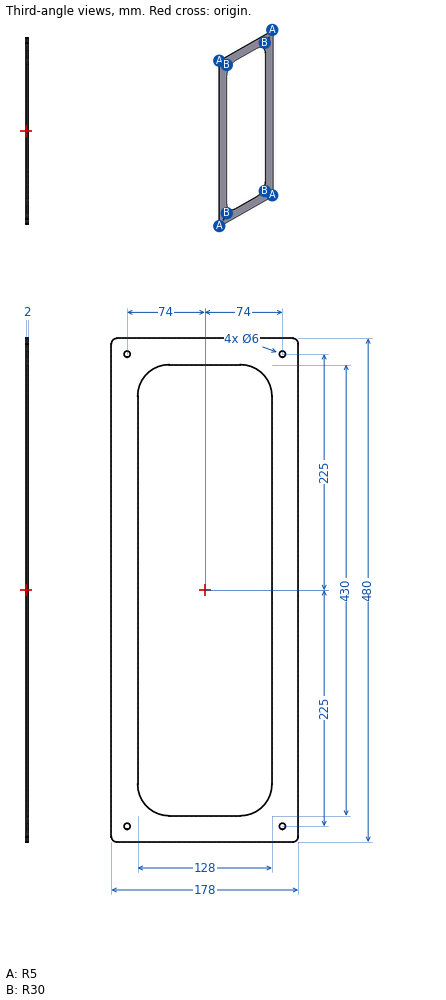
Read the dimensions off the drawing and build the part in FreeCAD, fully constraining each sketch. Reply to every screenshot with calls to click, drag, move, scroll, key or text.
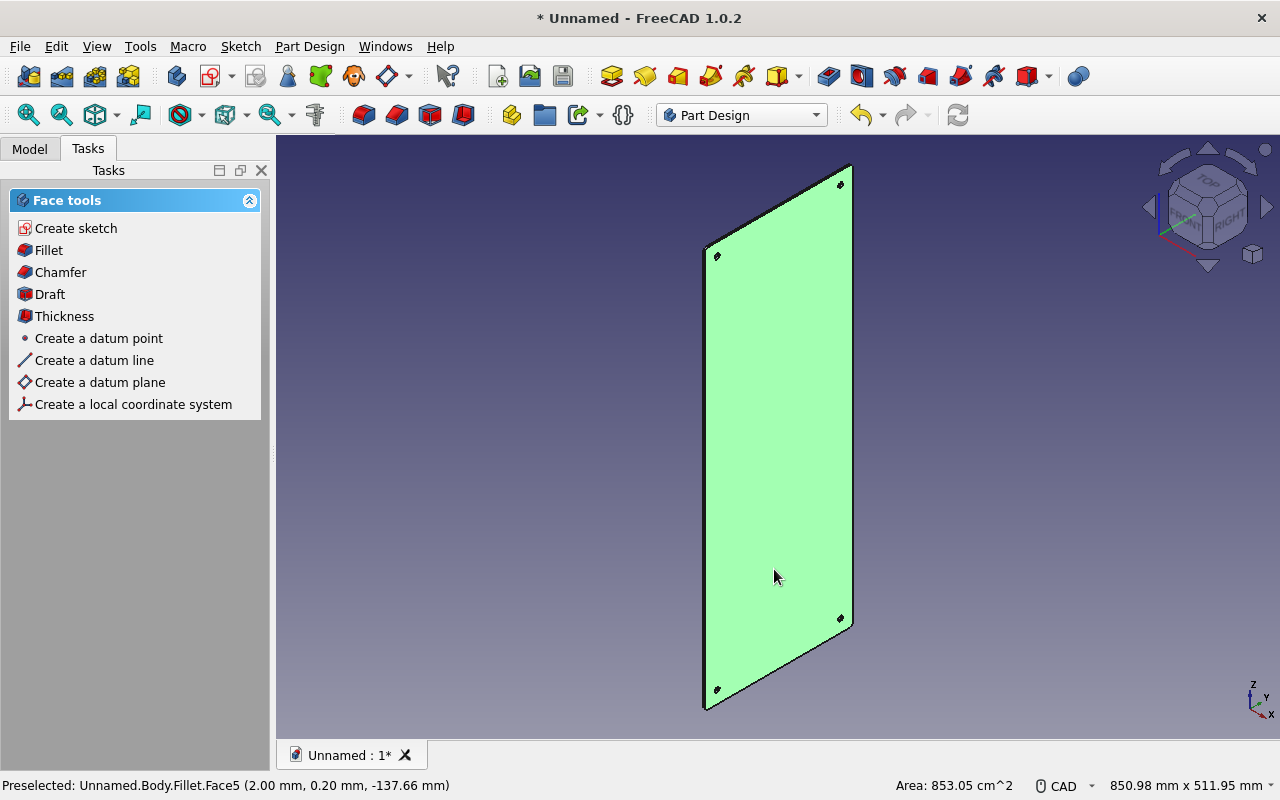
click(210, 76)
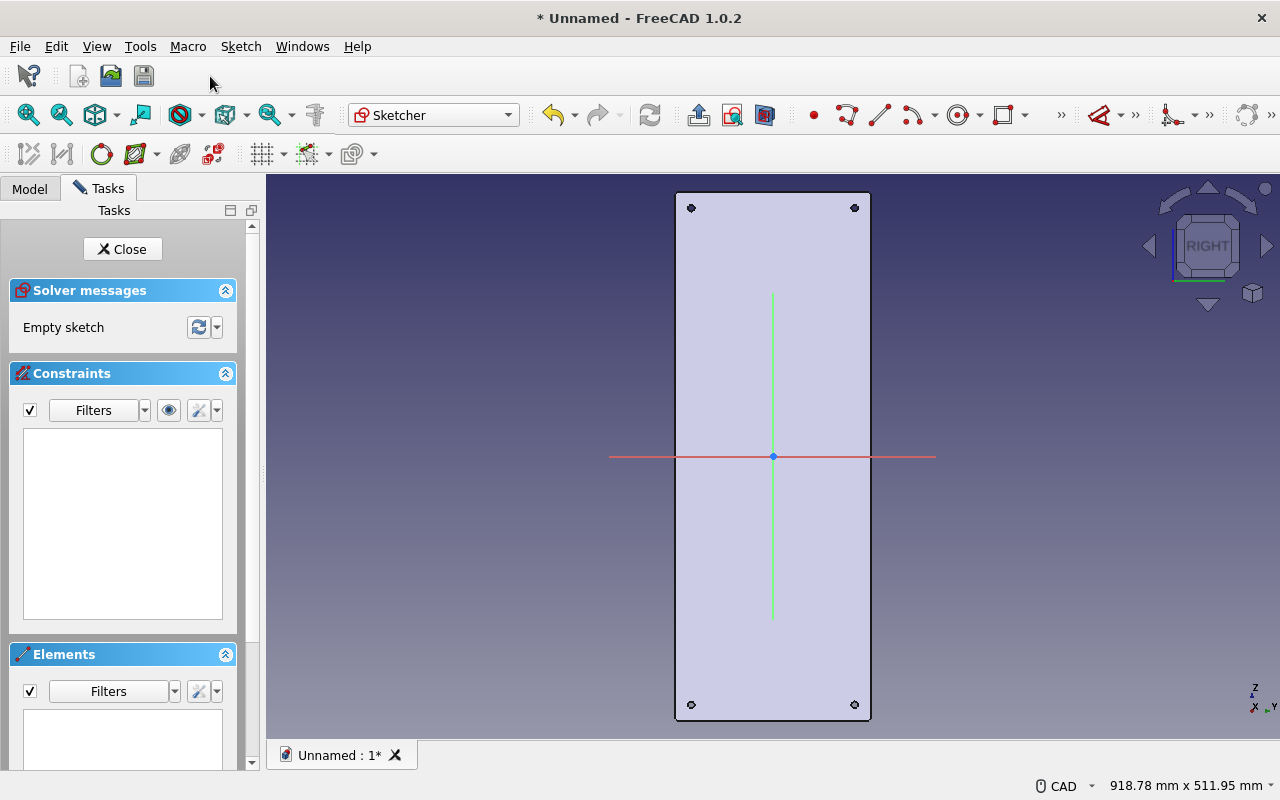
scroll(395, 456, down, 1)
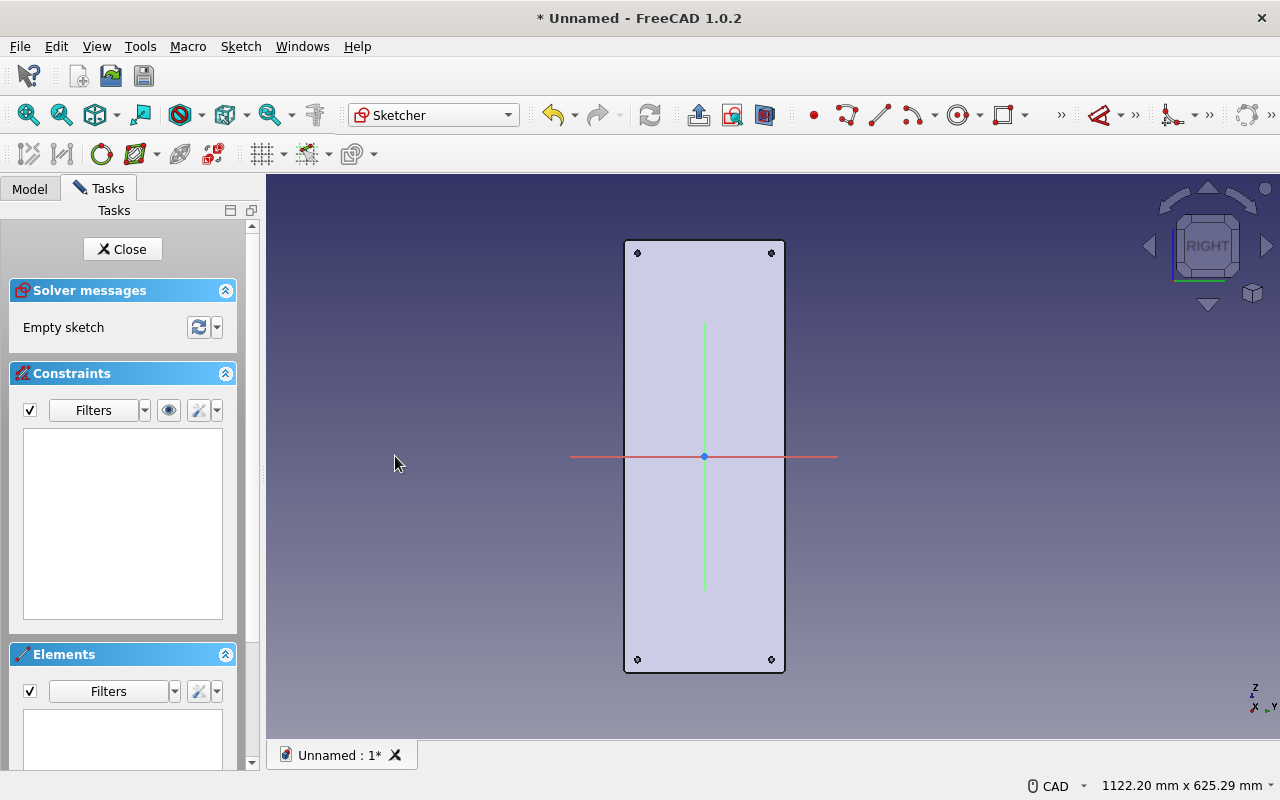
key(g)
key(v)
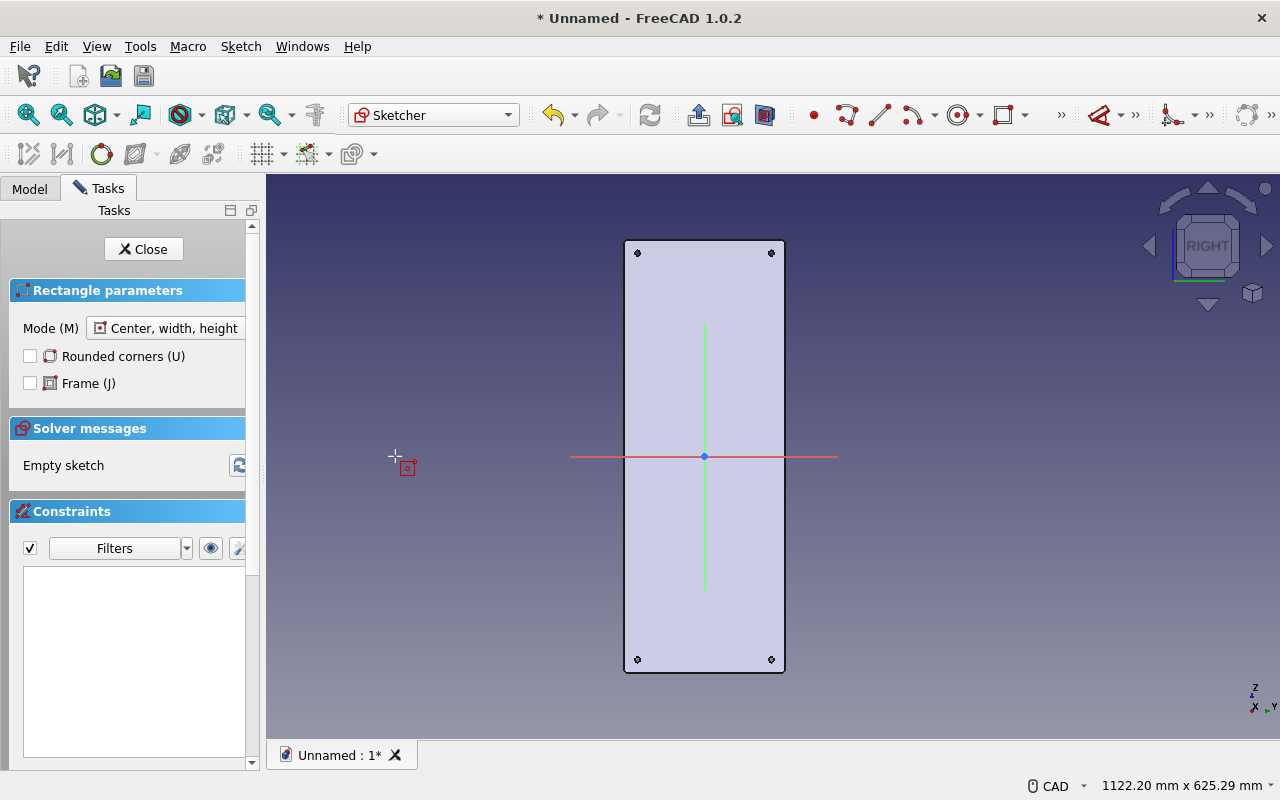
click(705, 456)
move(762, 262)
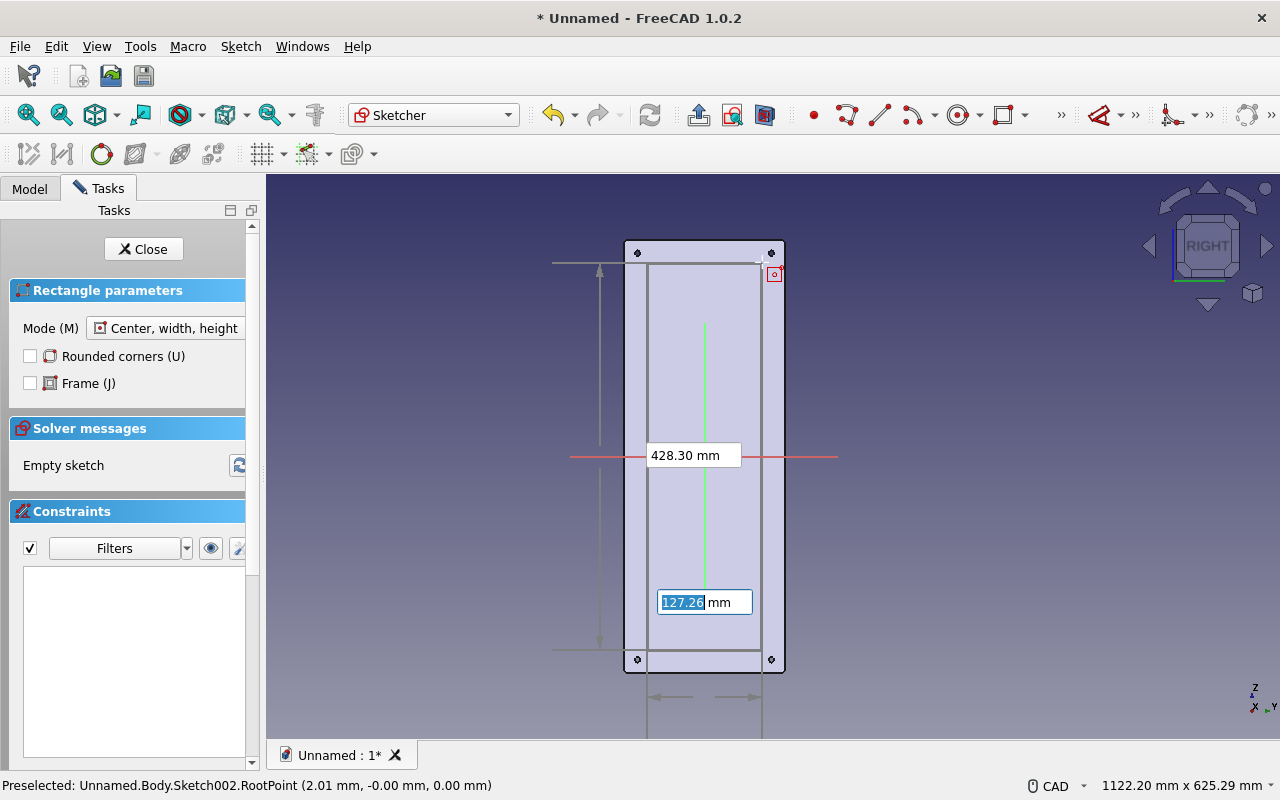
text(128)
key(Tab)
text(430)
key(Return)
key(Escape)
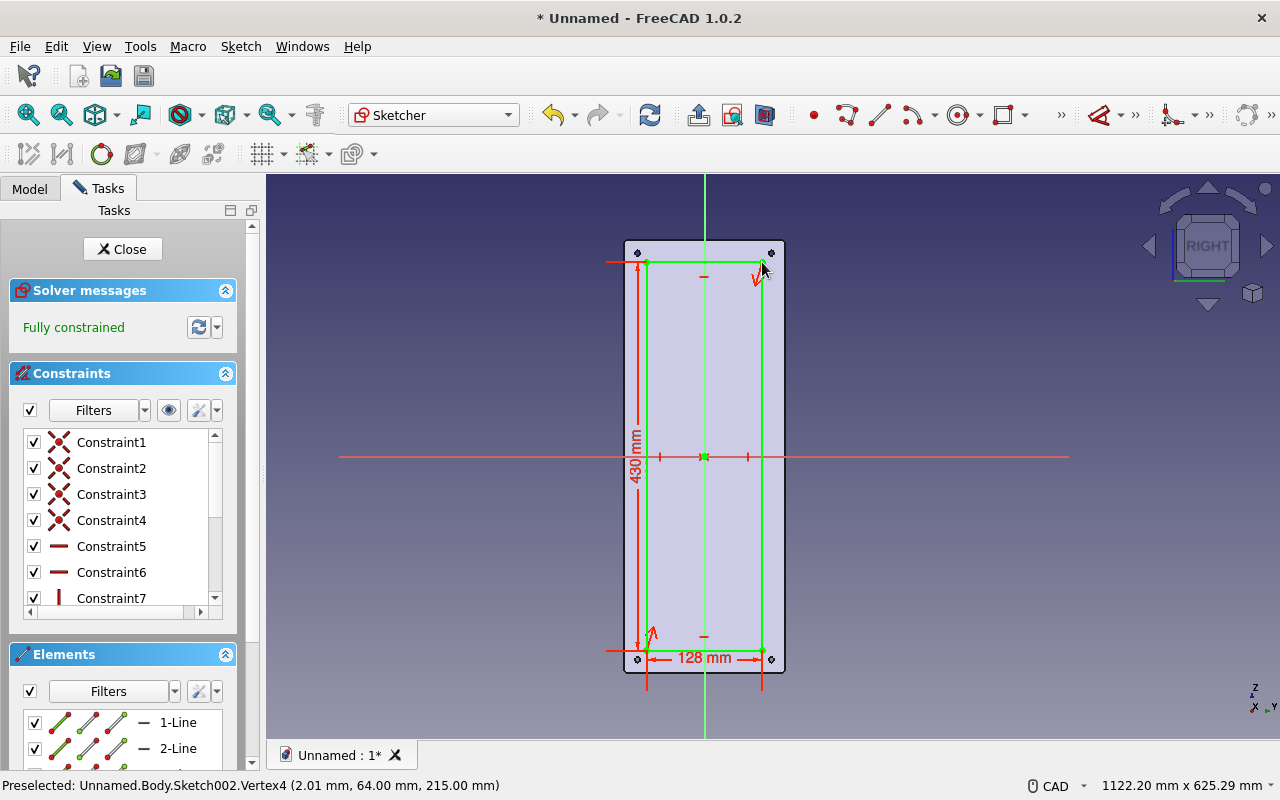
click(123, 249)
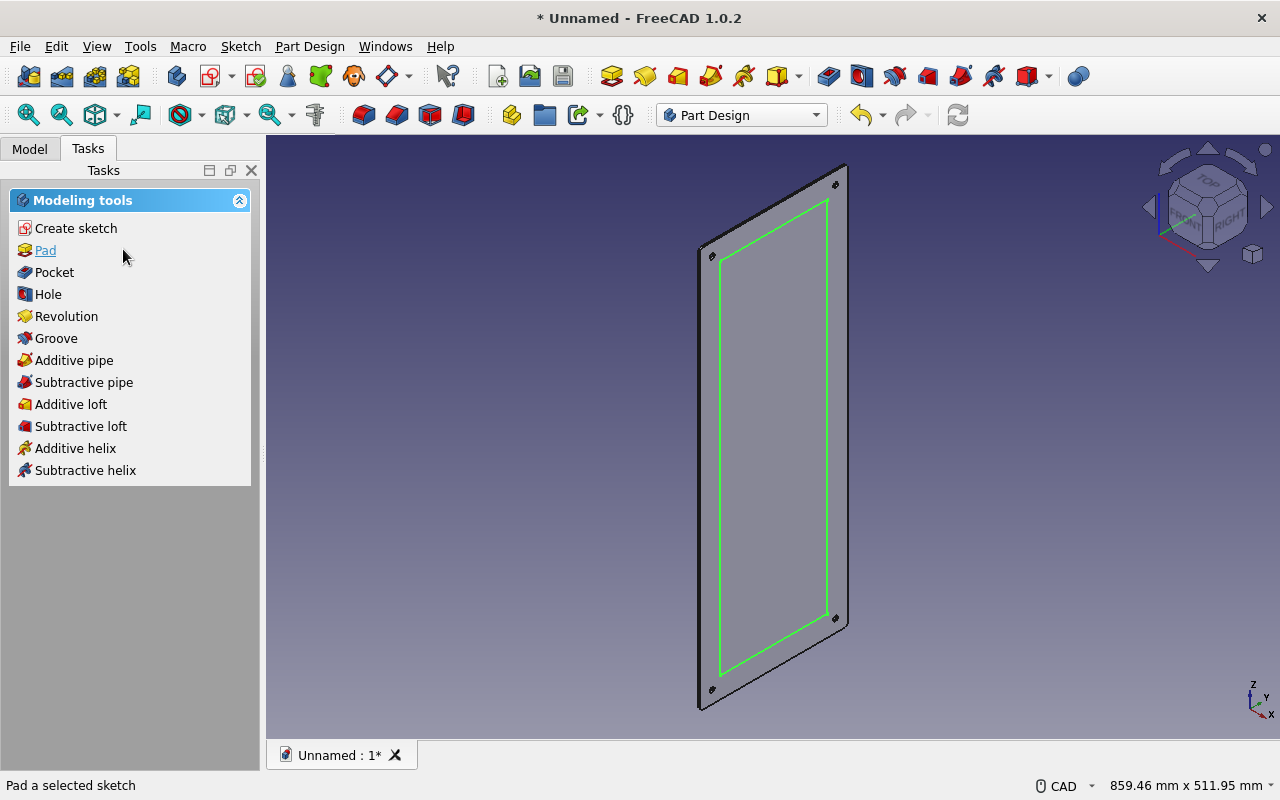
click(829, 76)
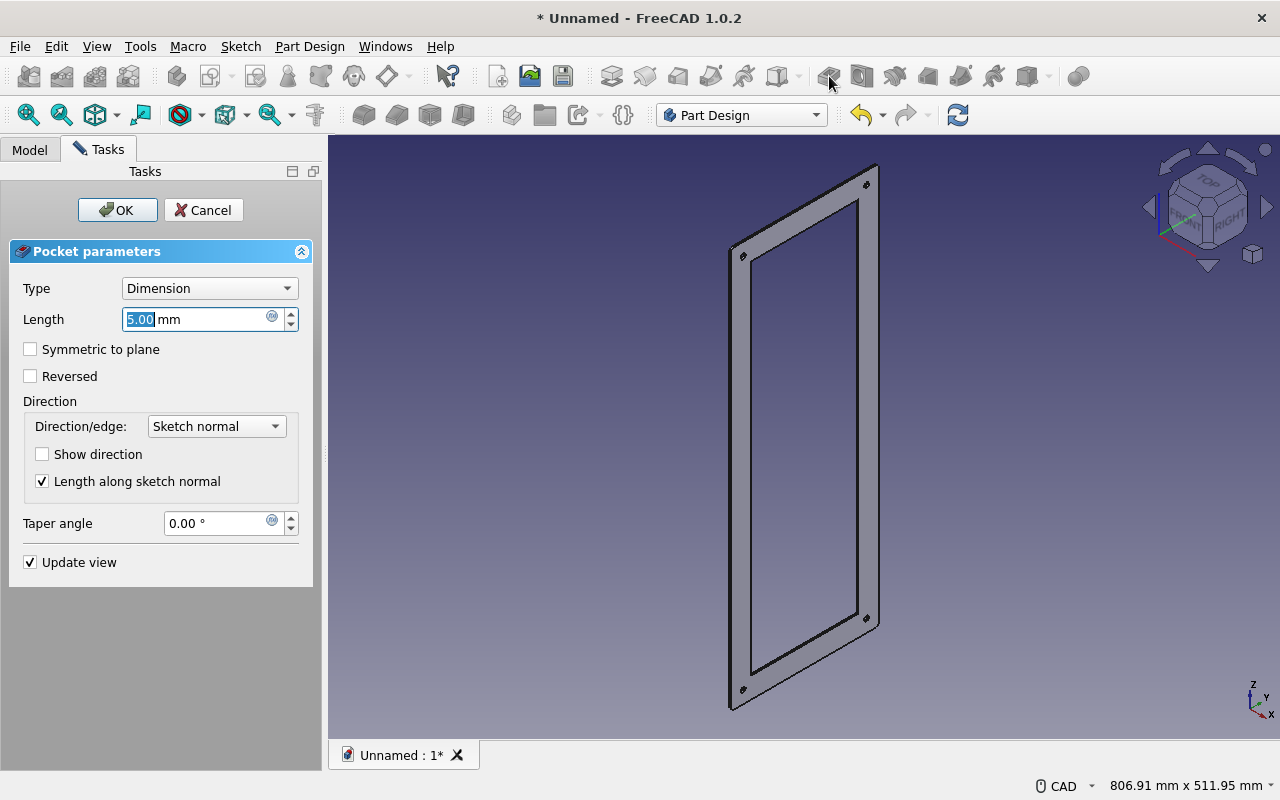
click(210, 288)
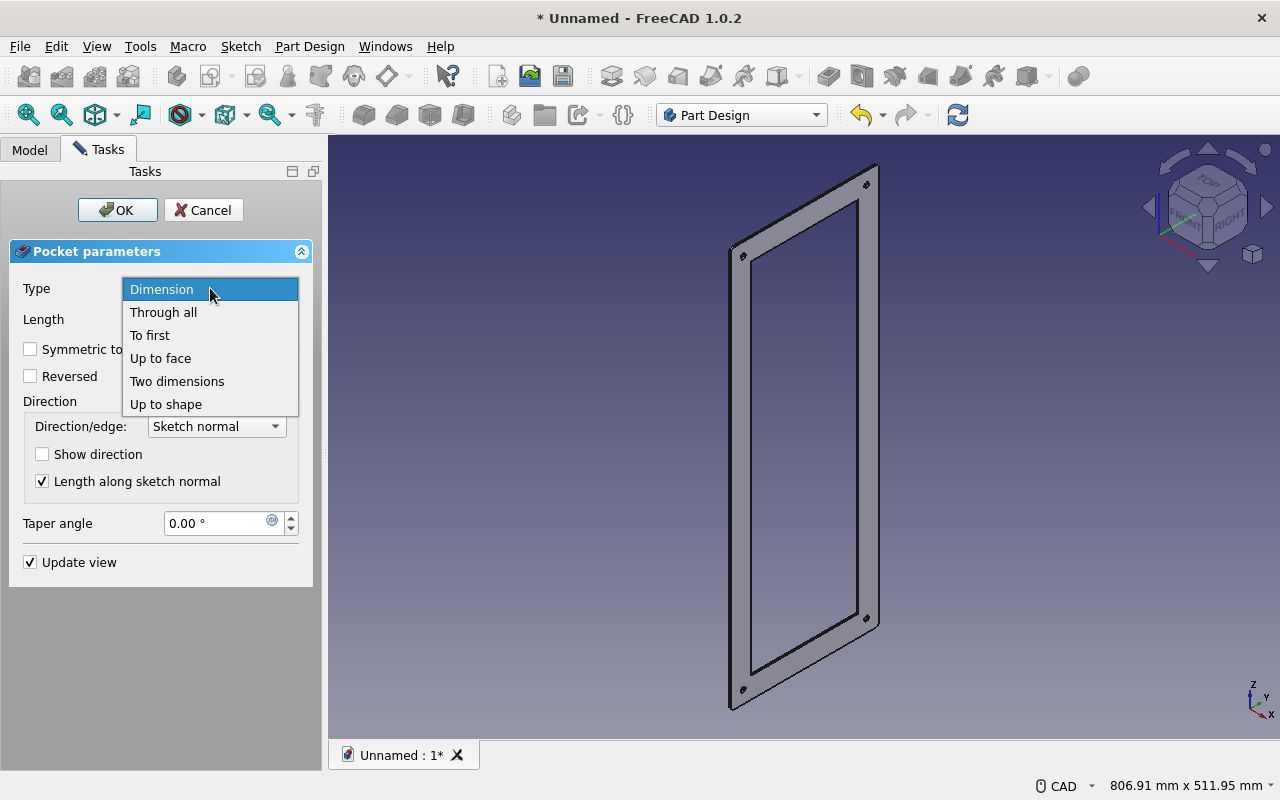
click(208, 312)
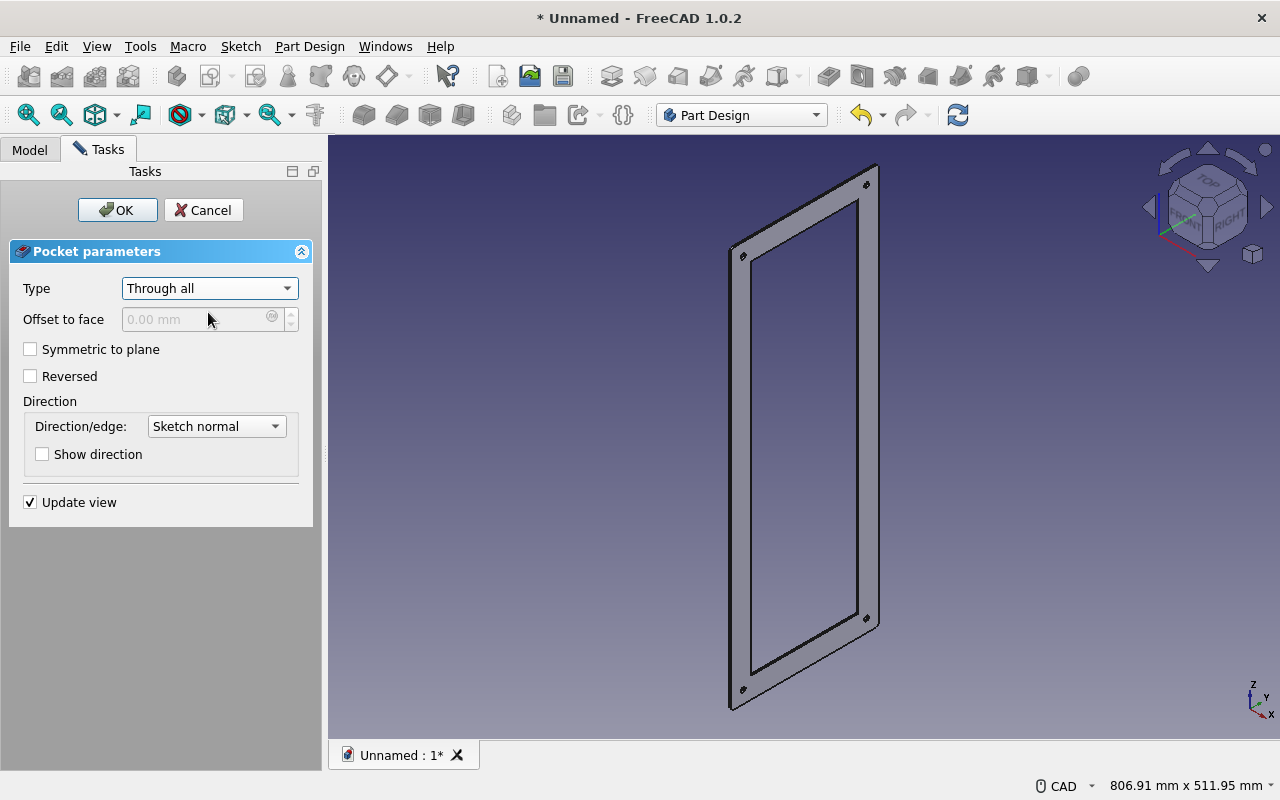
click(118, 210)